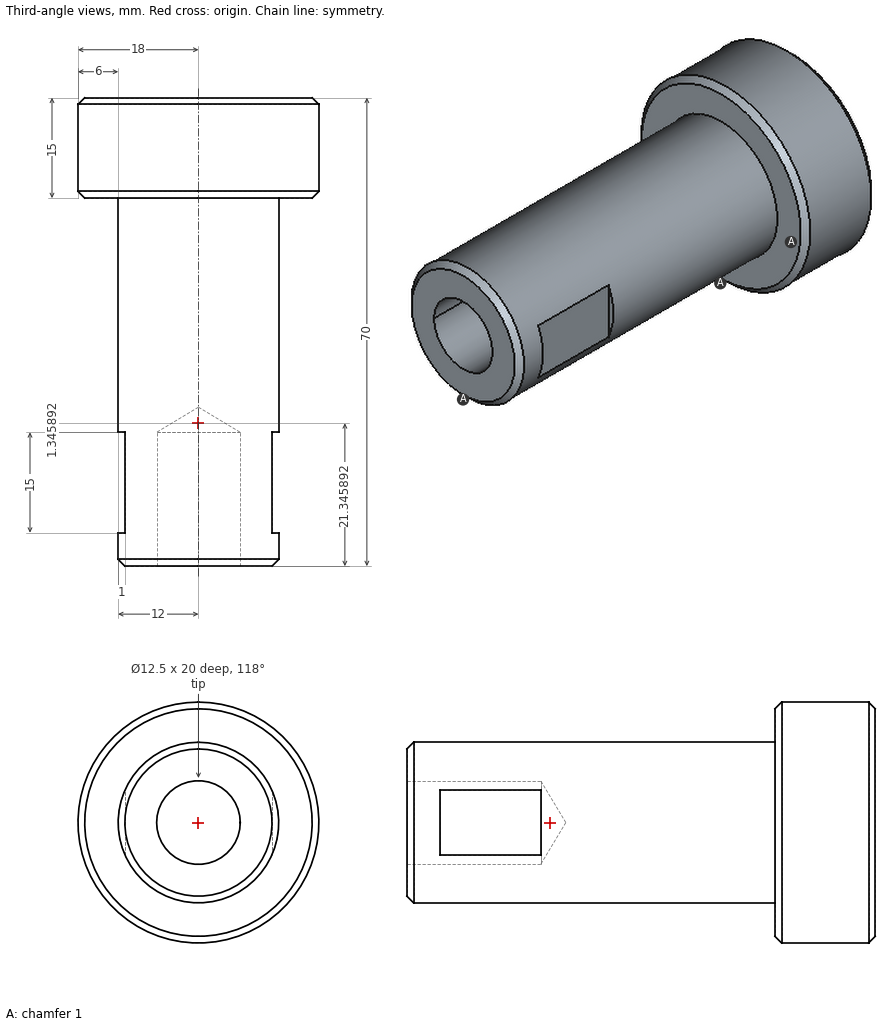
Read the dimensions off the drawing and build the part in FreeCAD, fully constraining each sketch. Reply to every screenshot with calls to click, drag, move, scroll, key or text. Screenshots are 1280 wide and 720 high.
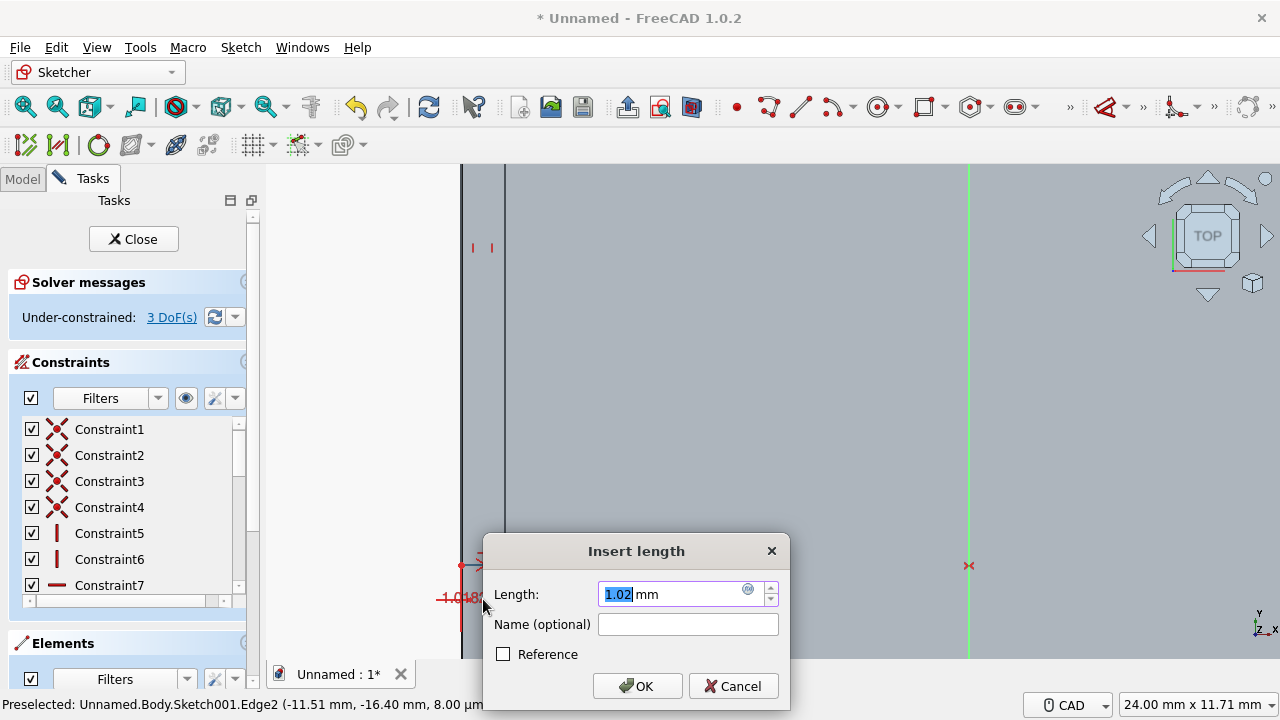
text(1)
key(Return)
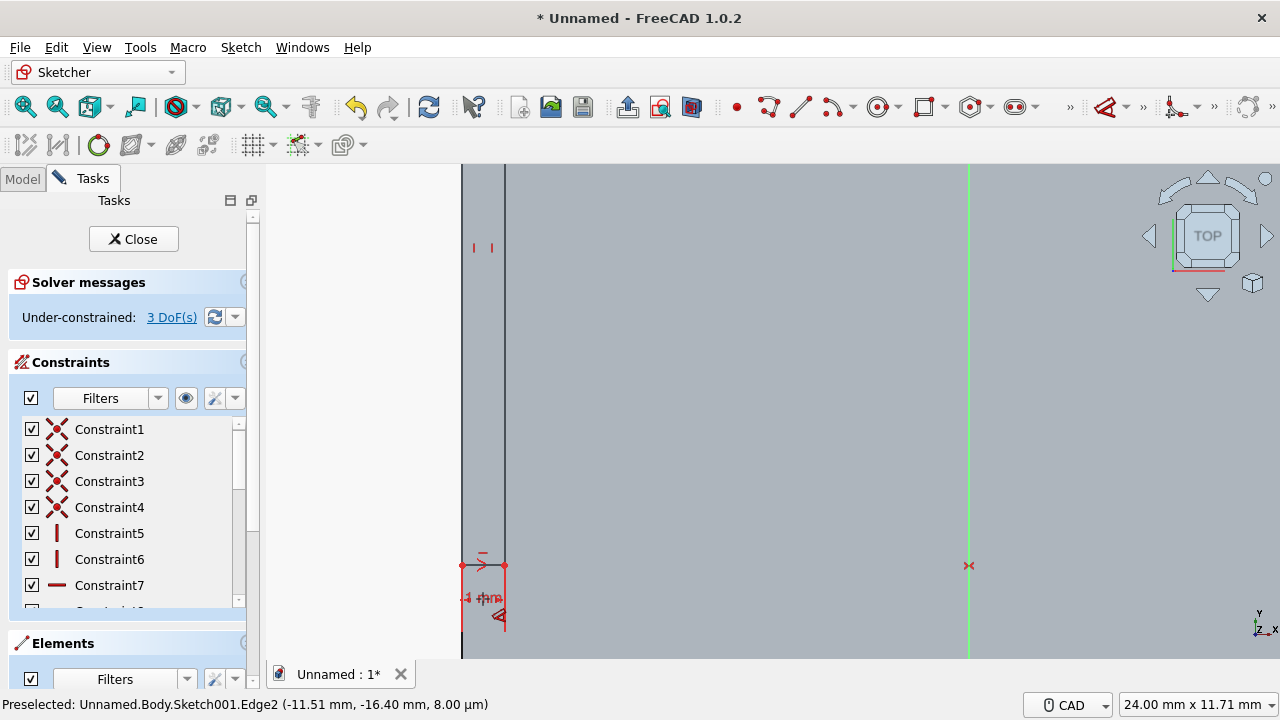
click(462, 375)
click(428, 379)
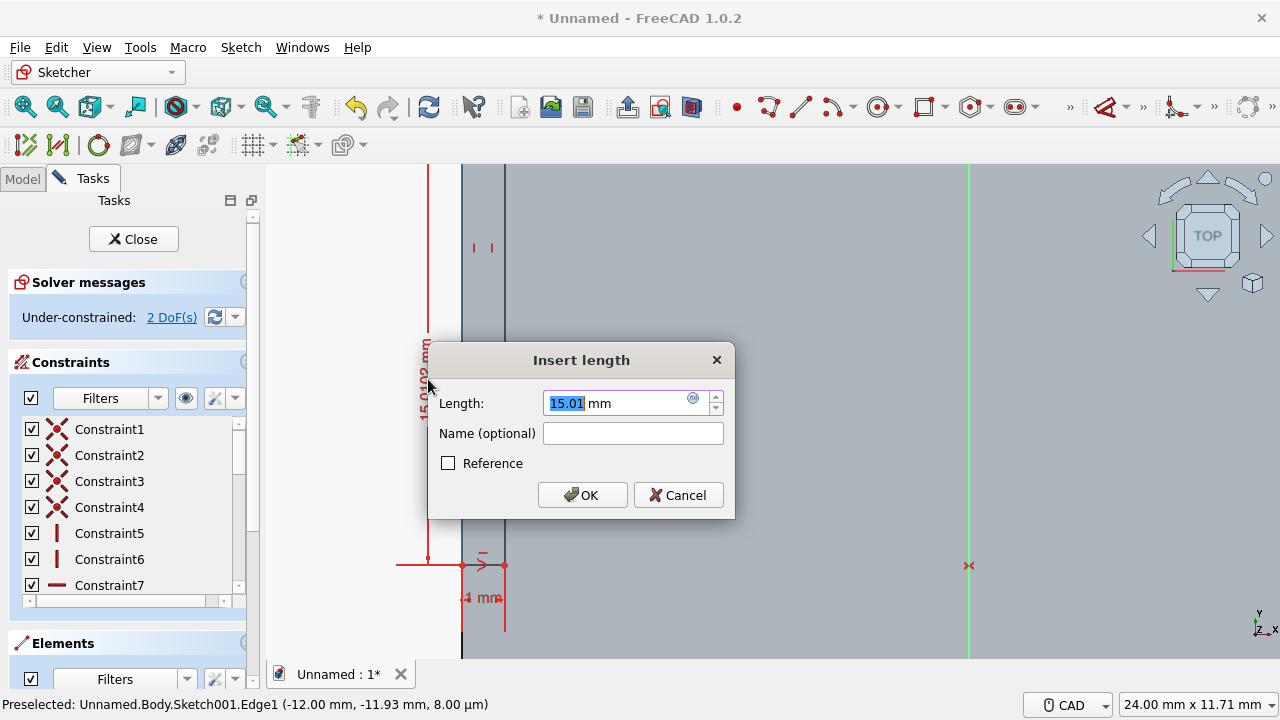
text(15)
key(Return)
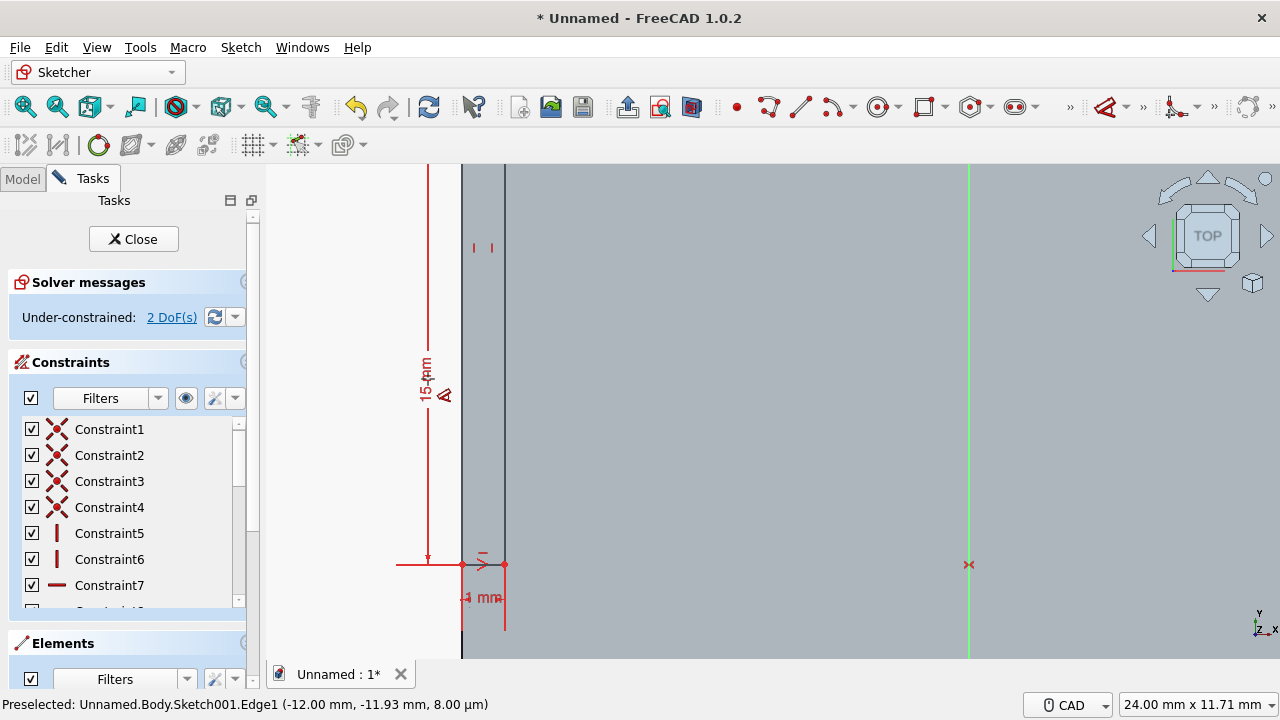
scroll(488, 570, down, 4)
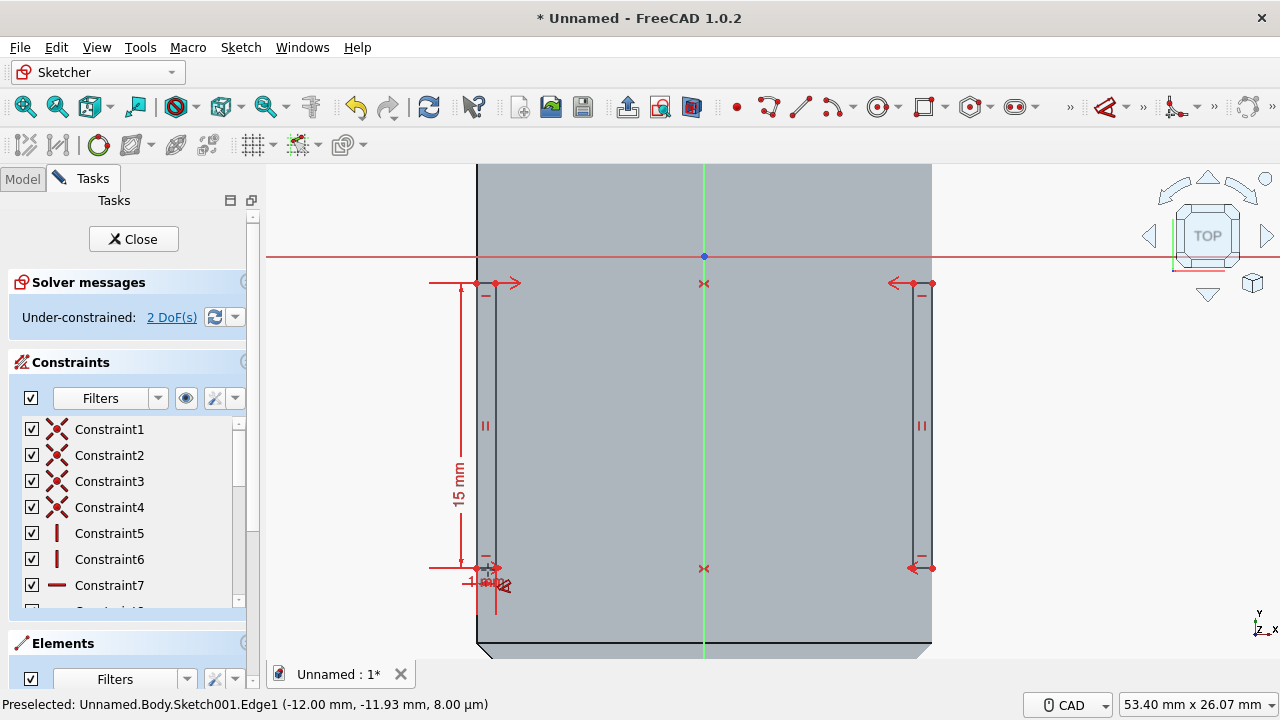
click(477, 283)
click(590, 223)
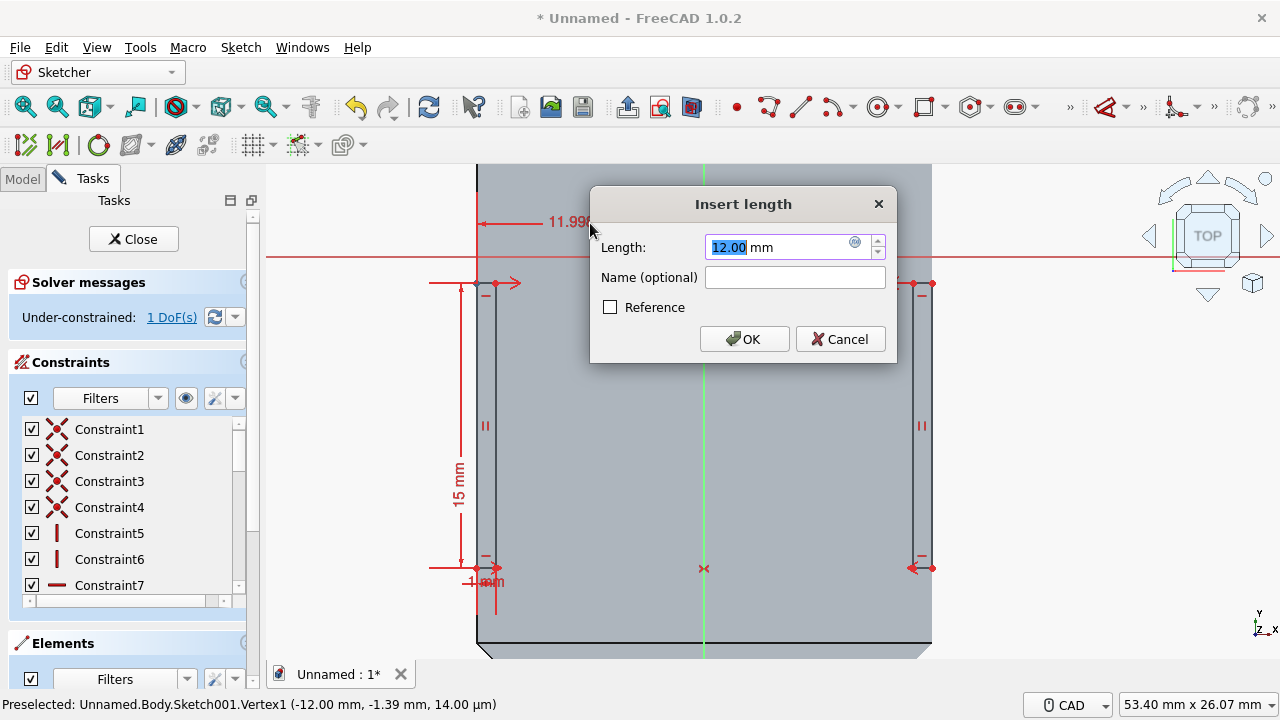
text(12)
key(Return)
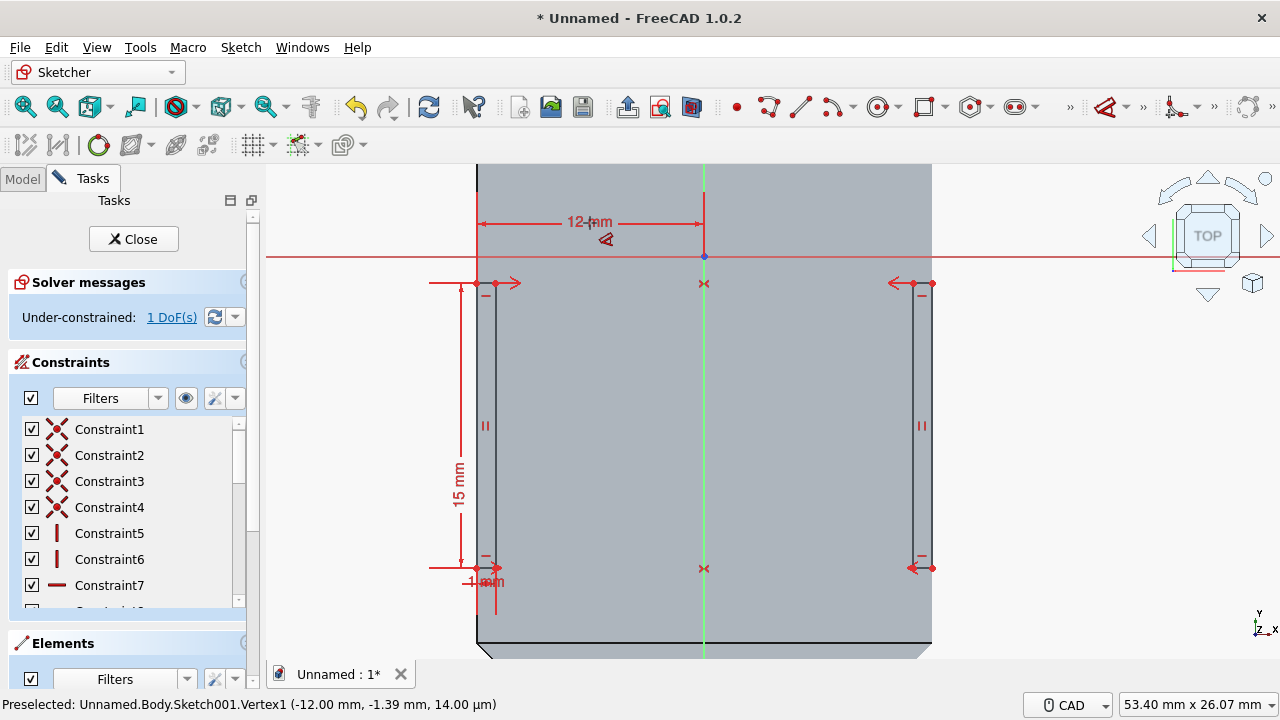
scroll(477, 283, up, 3)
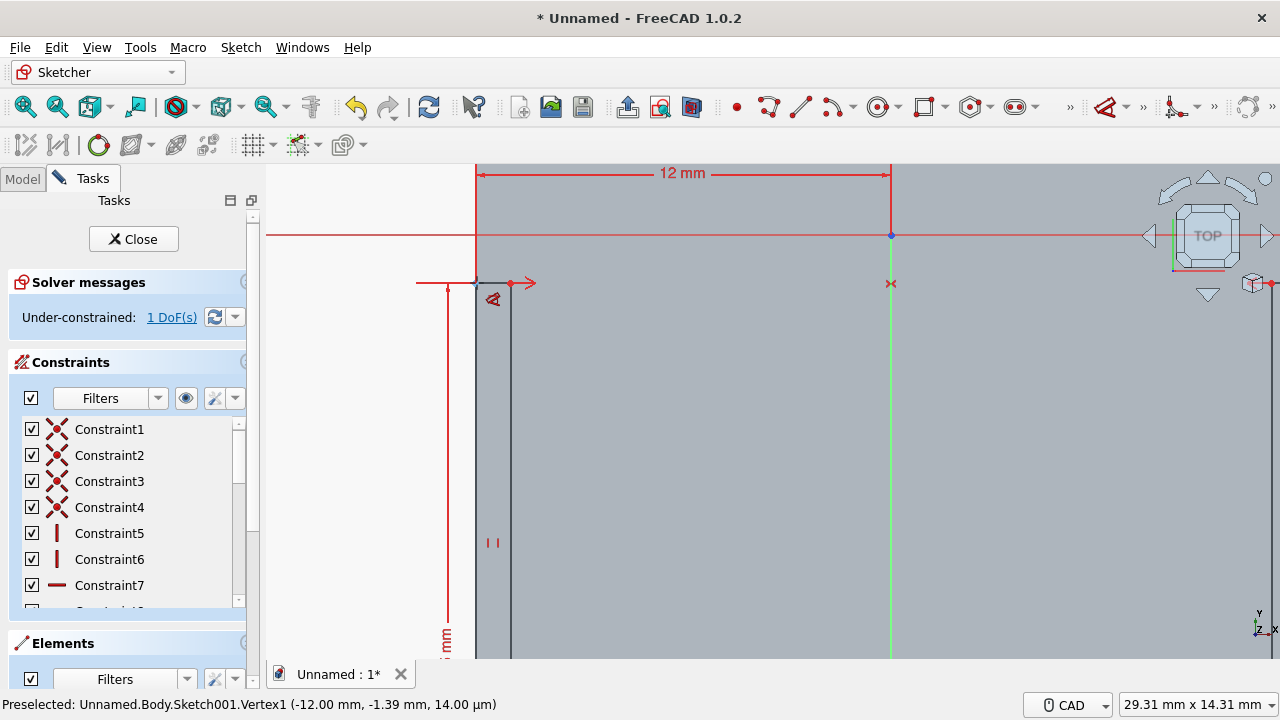
click(476, 283)
click(442, 259)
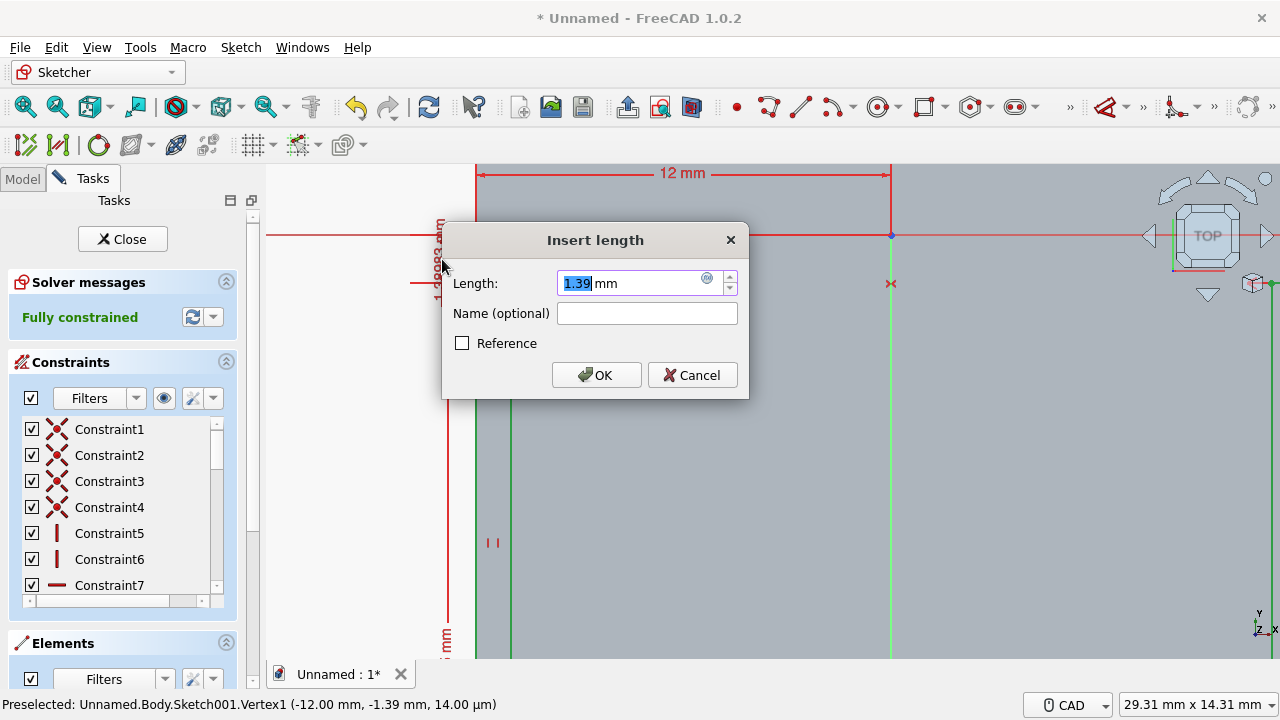
text(1.345892)
key(Return)
key(Escape)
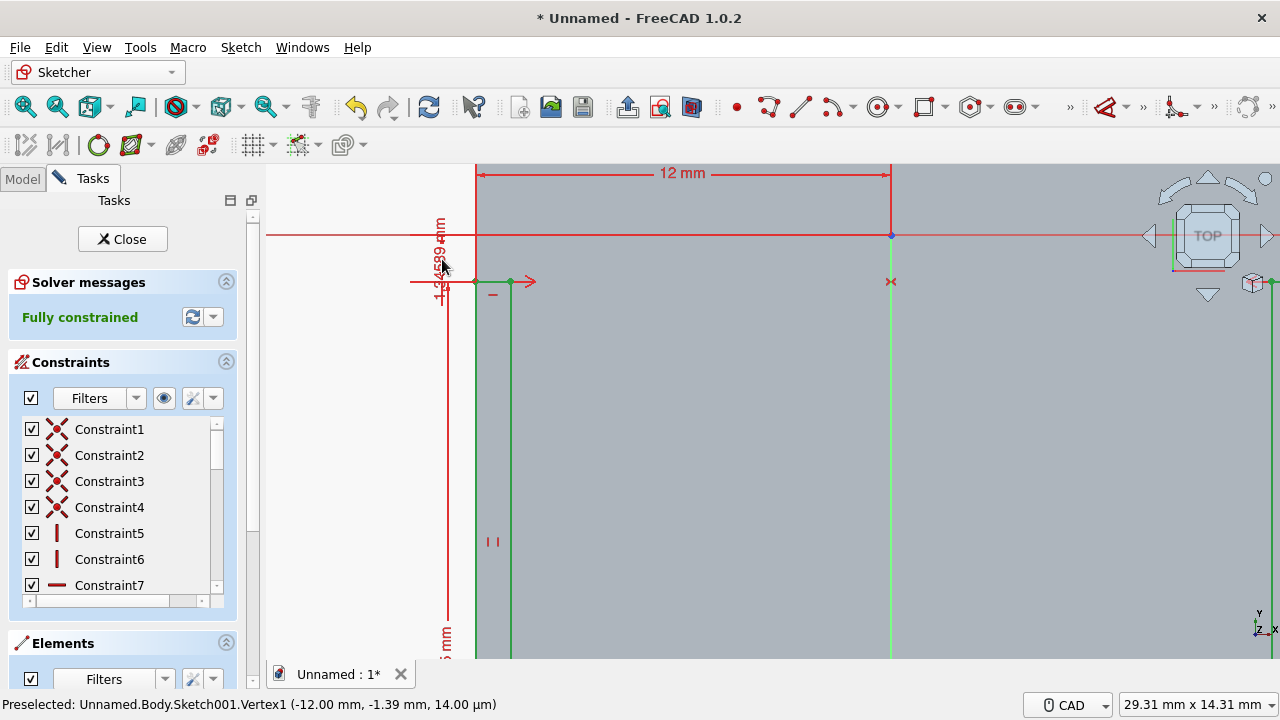
click(123, 239)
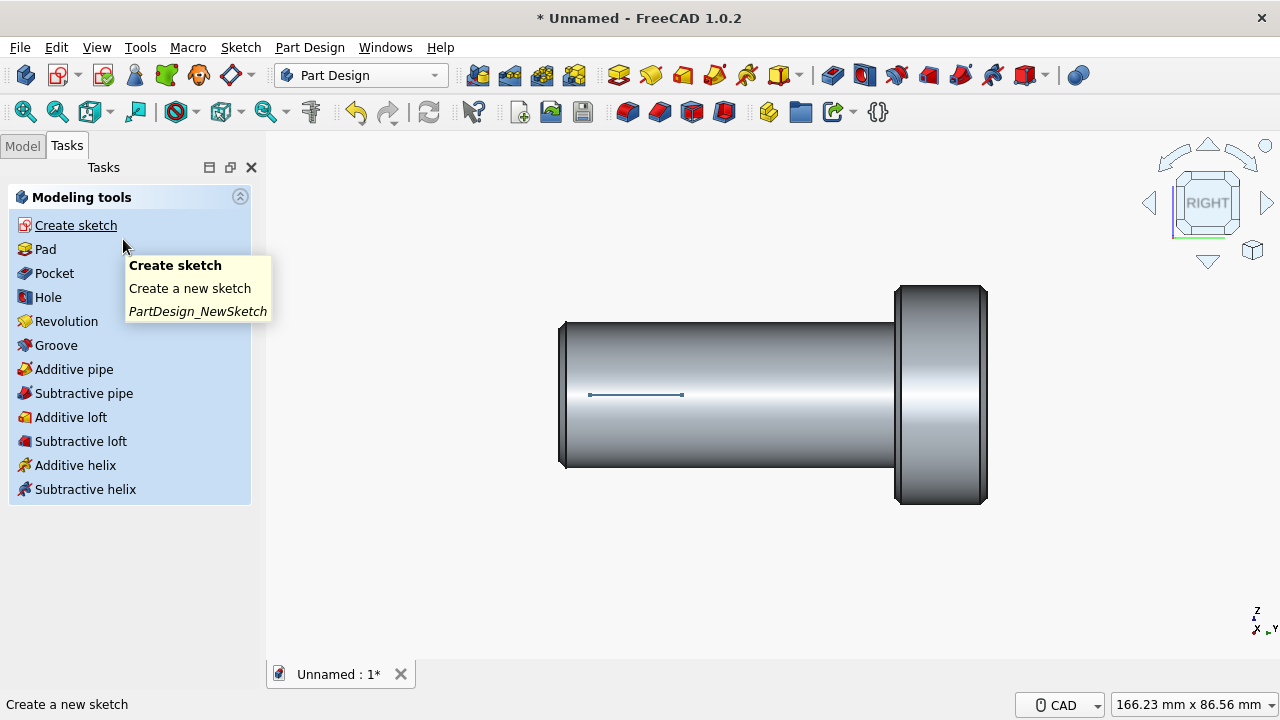
click(834, 76)